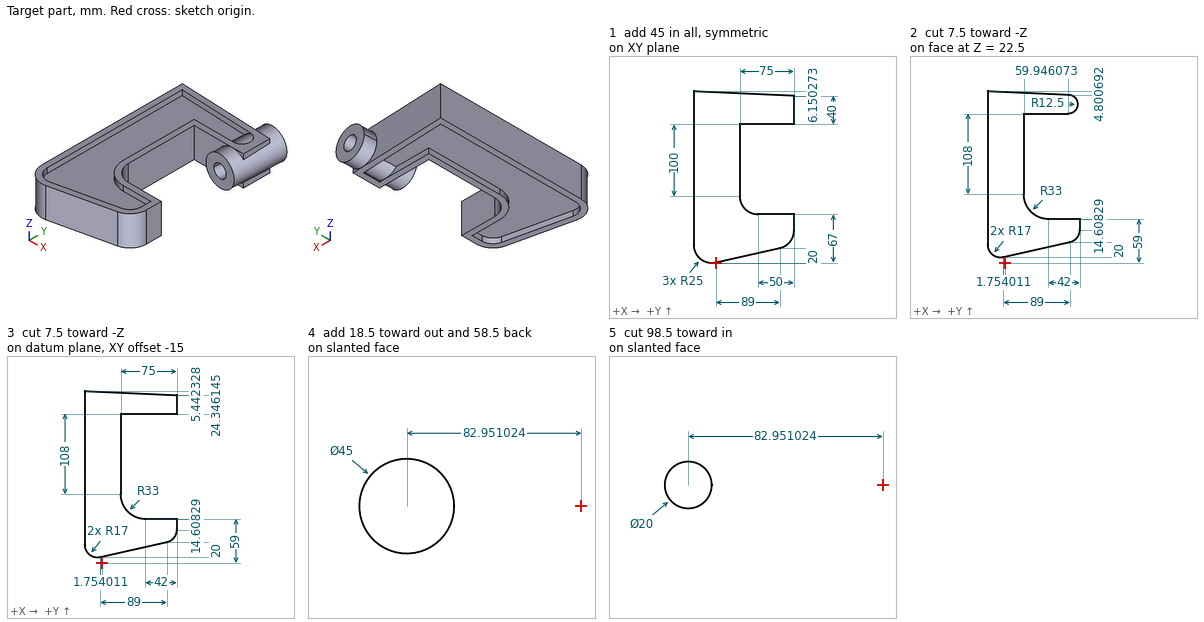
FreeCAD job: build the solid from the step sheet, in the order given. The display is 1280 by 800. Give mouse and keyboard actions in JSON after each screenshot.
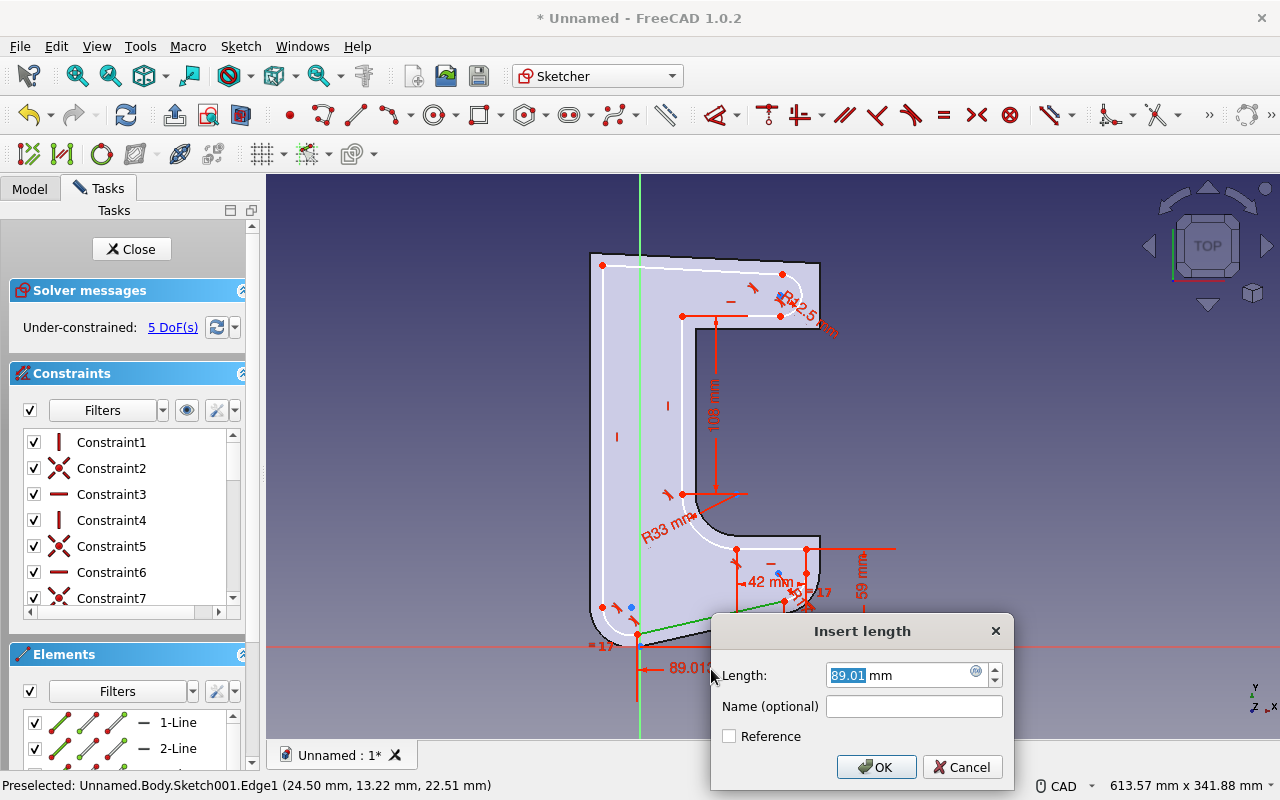
{"action": "type", "text": "89"}
{"action": "key", "text": "Return"}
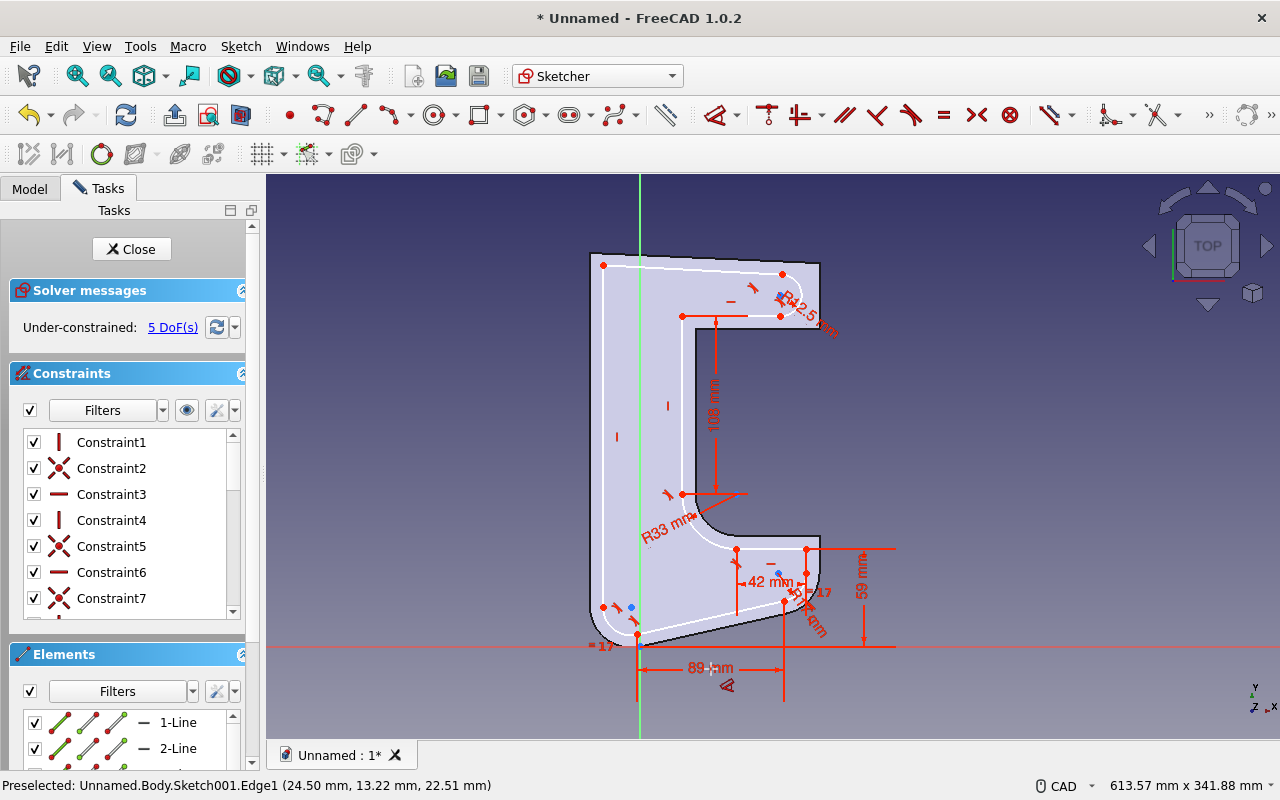
{"action": "left_click", "coordinate": [681, 625]}
{"action": "left_click", "coordinate": [579, 618]}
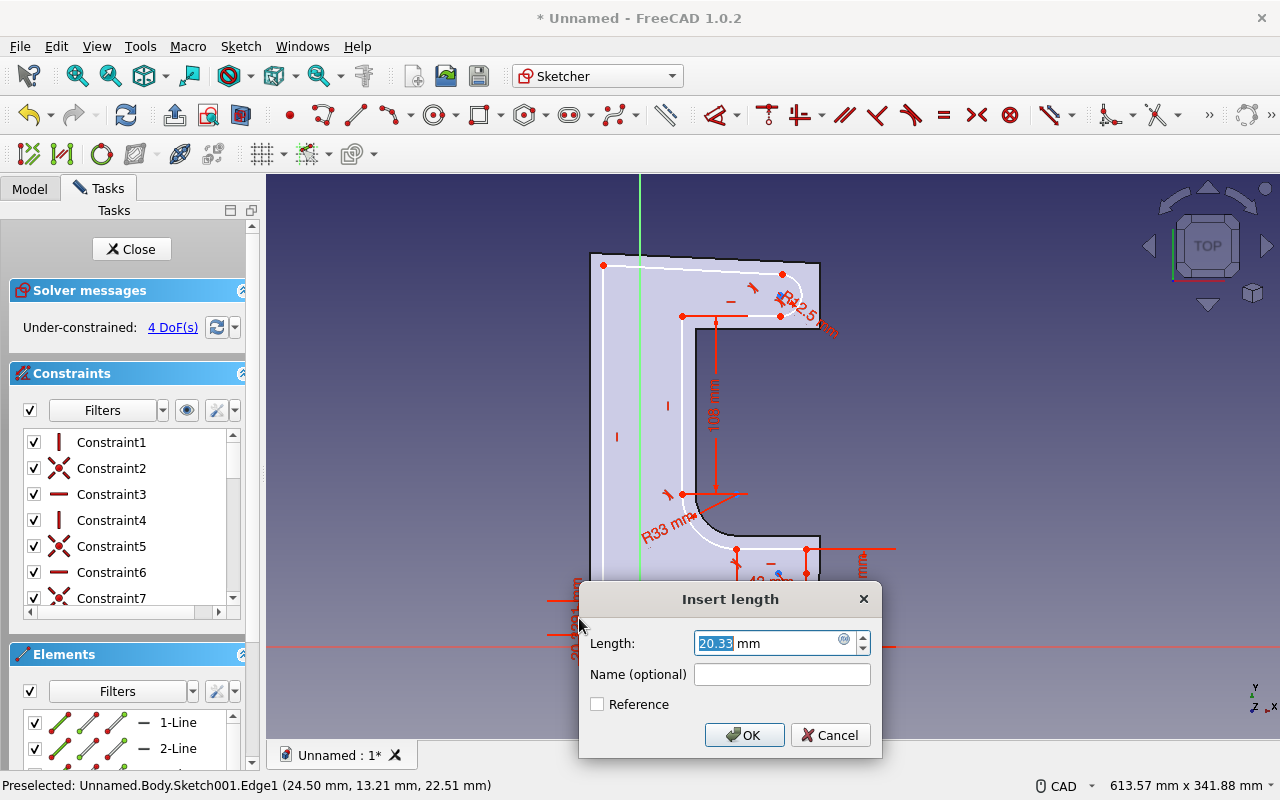
{"action": "type", "text": "20"}
{"action": "key", "text": "Return"}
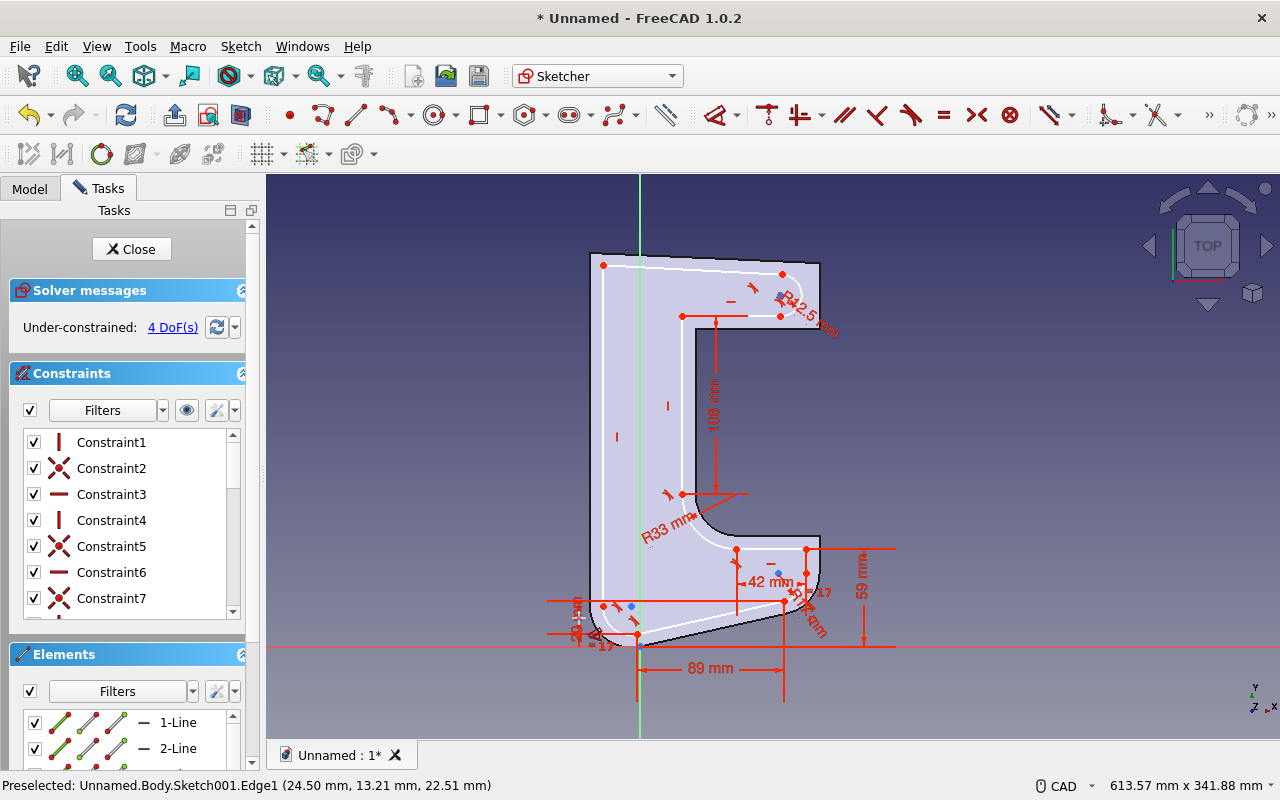
{"action": "scroll", "coordinate": [806, 564], "scroll_direction": "up", "scroll_amount": 3}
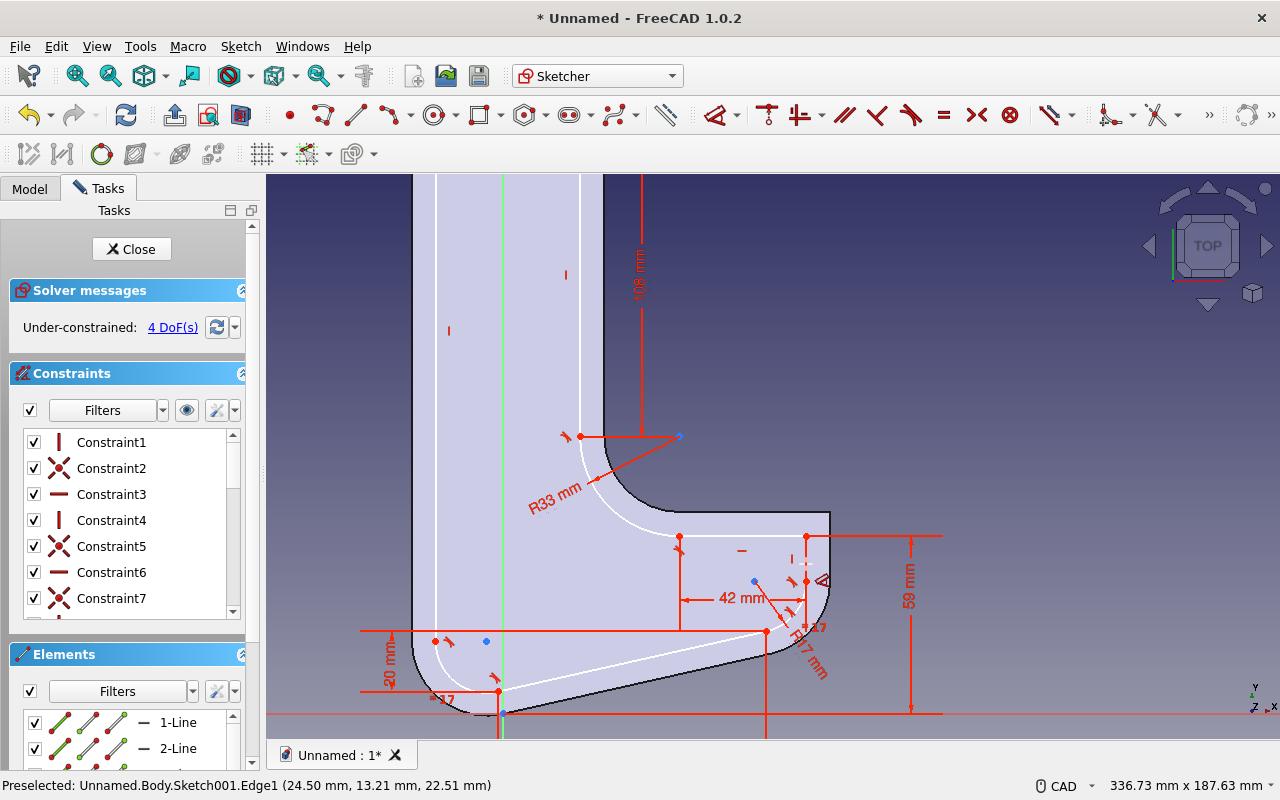
{"action": "left_click", "coordinate": [806, 563]}
{"action": "left_click", "coordinate": [840, 559]}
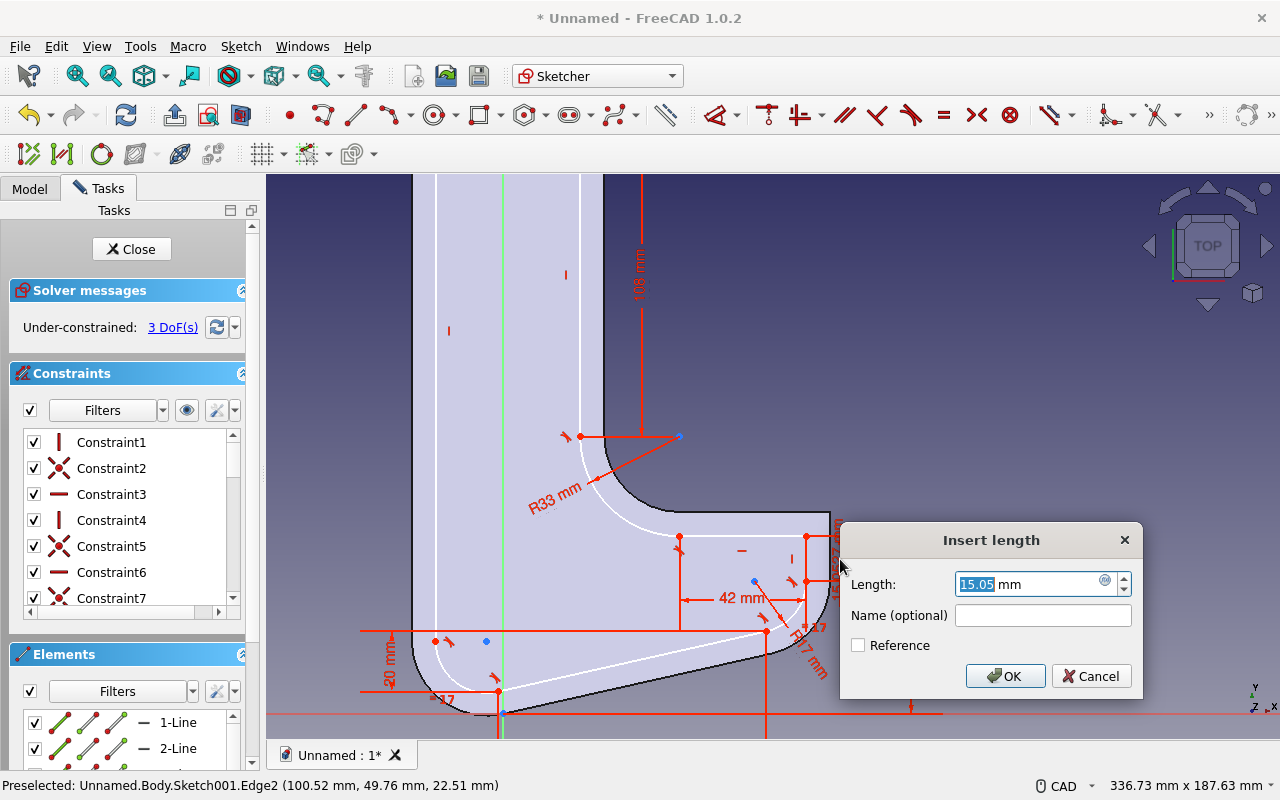
{"action": "type", "text": "14.60829"}
{"action": "key", "text": "Return"}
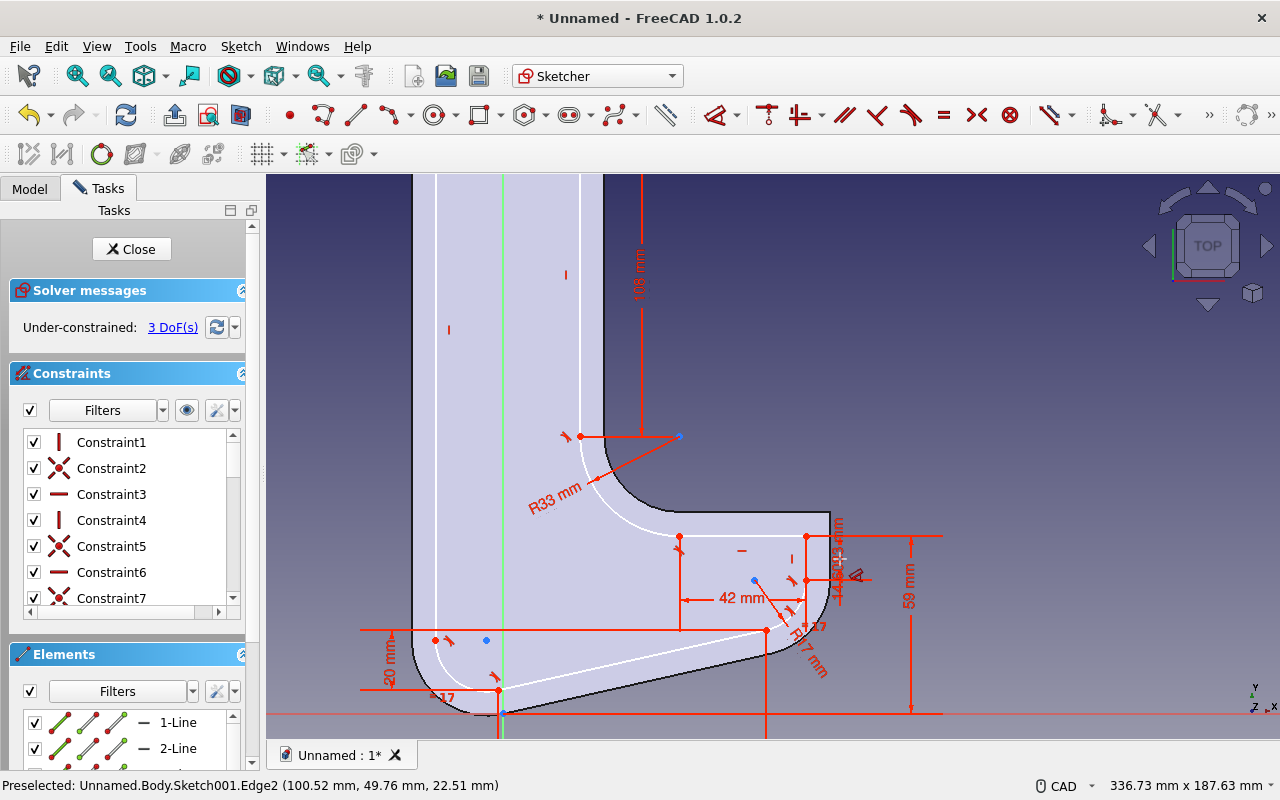
{"action": "scroll", "coordinate": [806, 564], "scroll_direction": "down", "scroll_amount": 3}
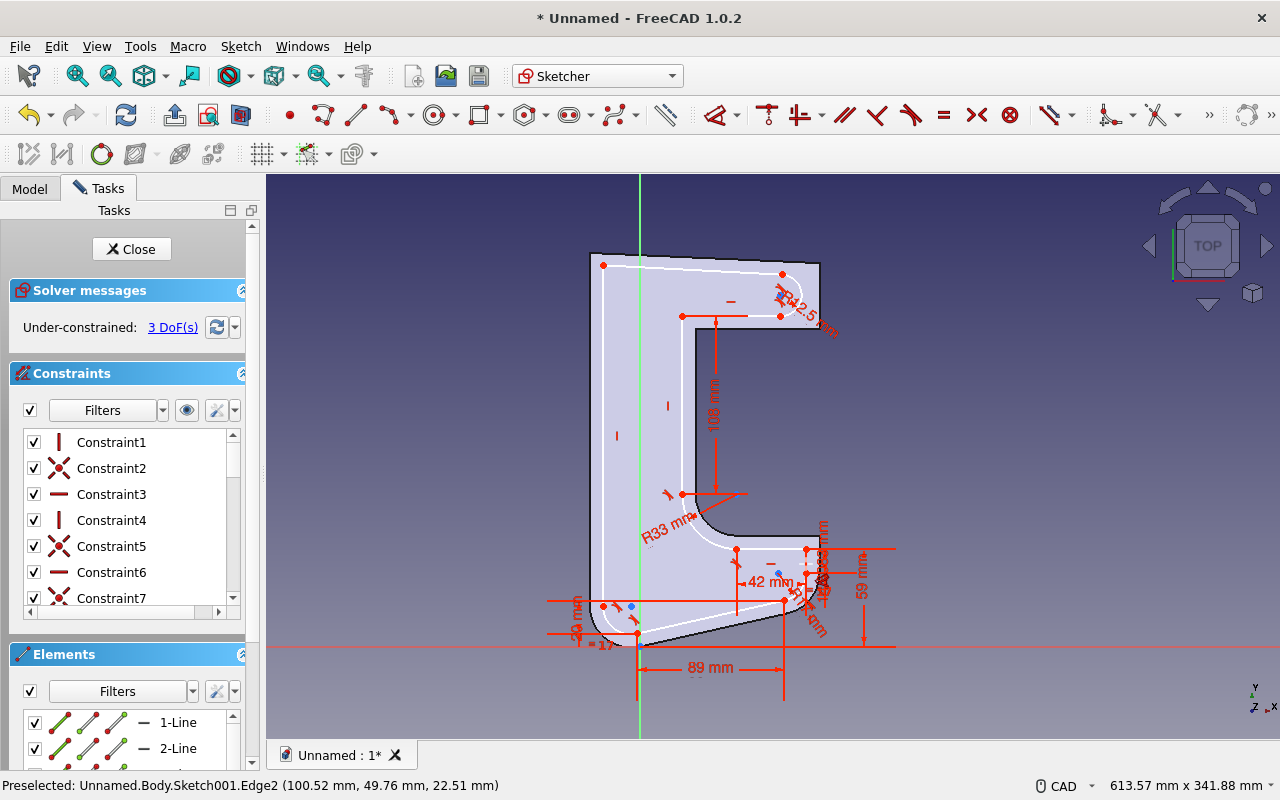
{"action": "left_click", "coordinate": [712, 316]}
{"action": "left_click", "coordinate": [732, 350]}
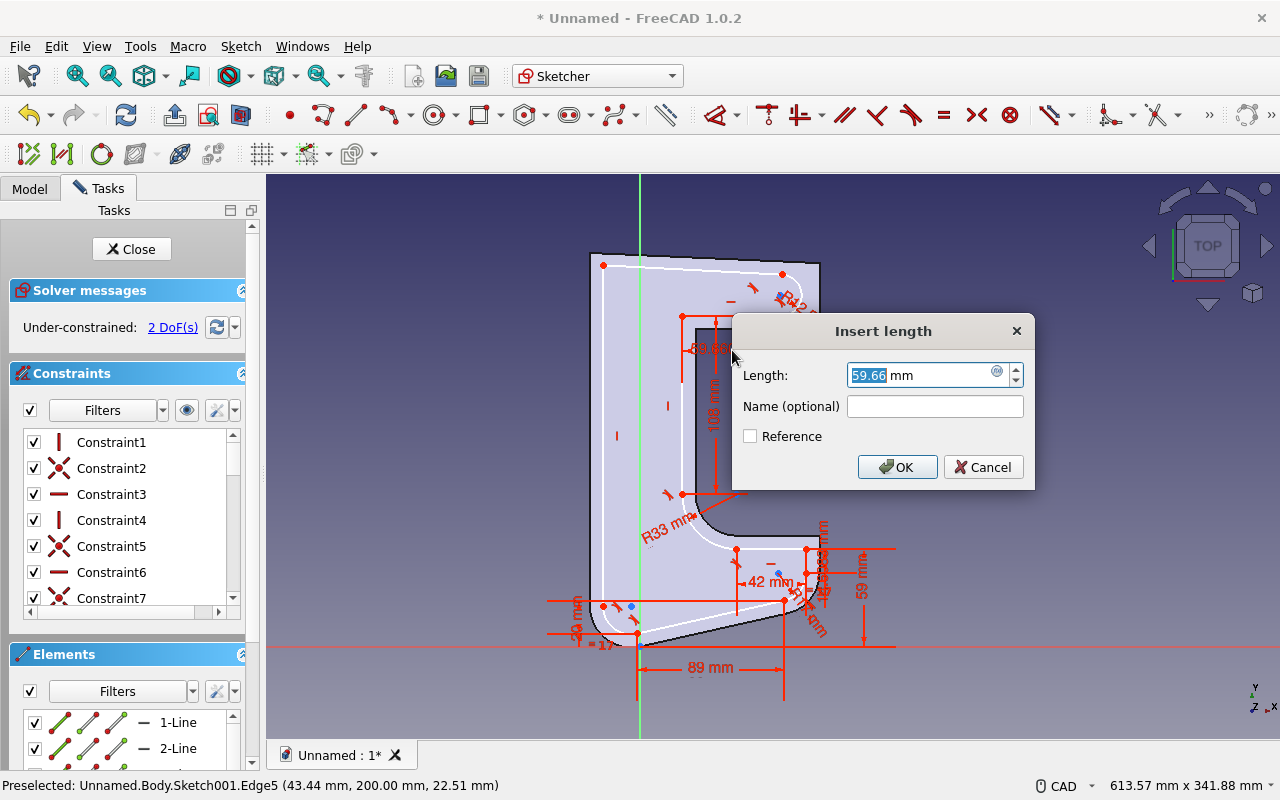
{"action": "type", "text": "59.946073"}
{"action": "key", "text": "Return"}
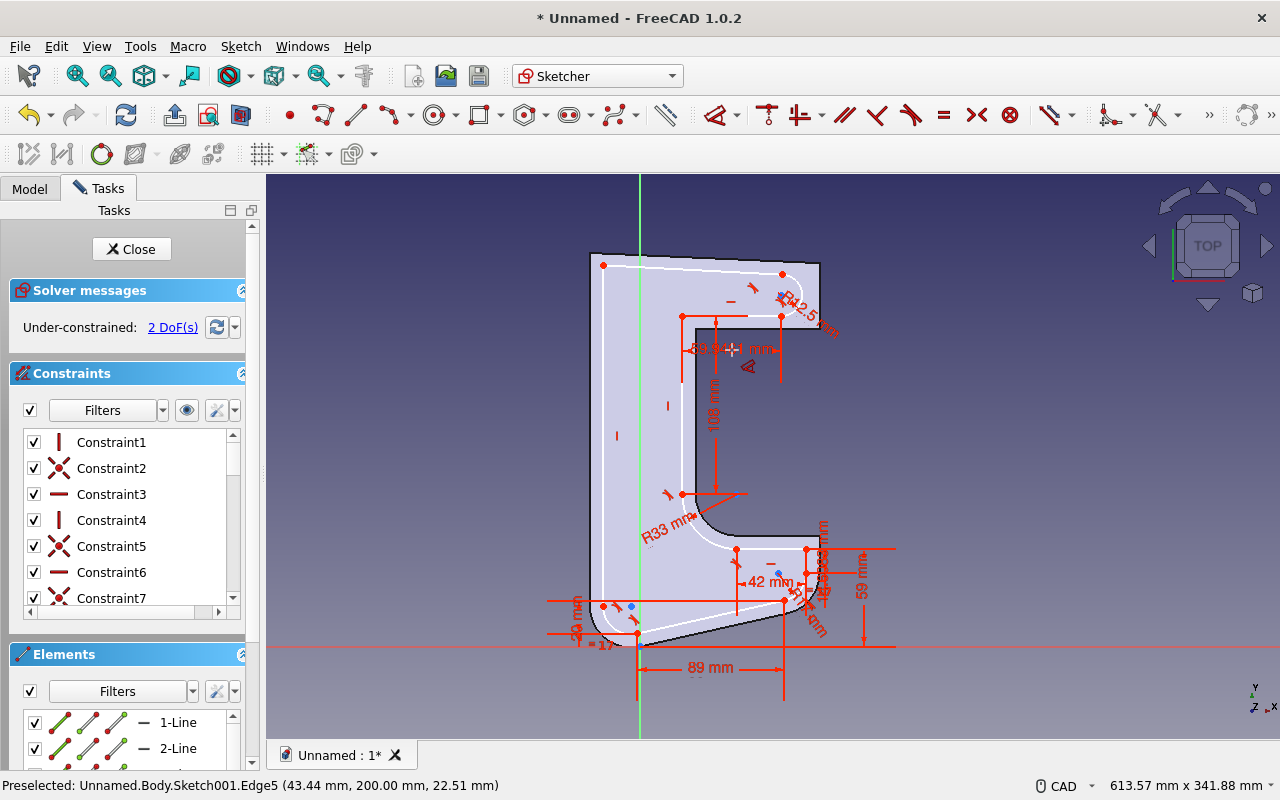
{"action": "scroll", "coordinate": [637, 634], "scroll_direction": "up", "scroll_amount": 14}